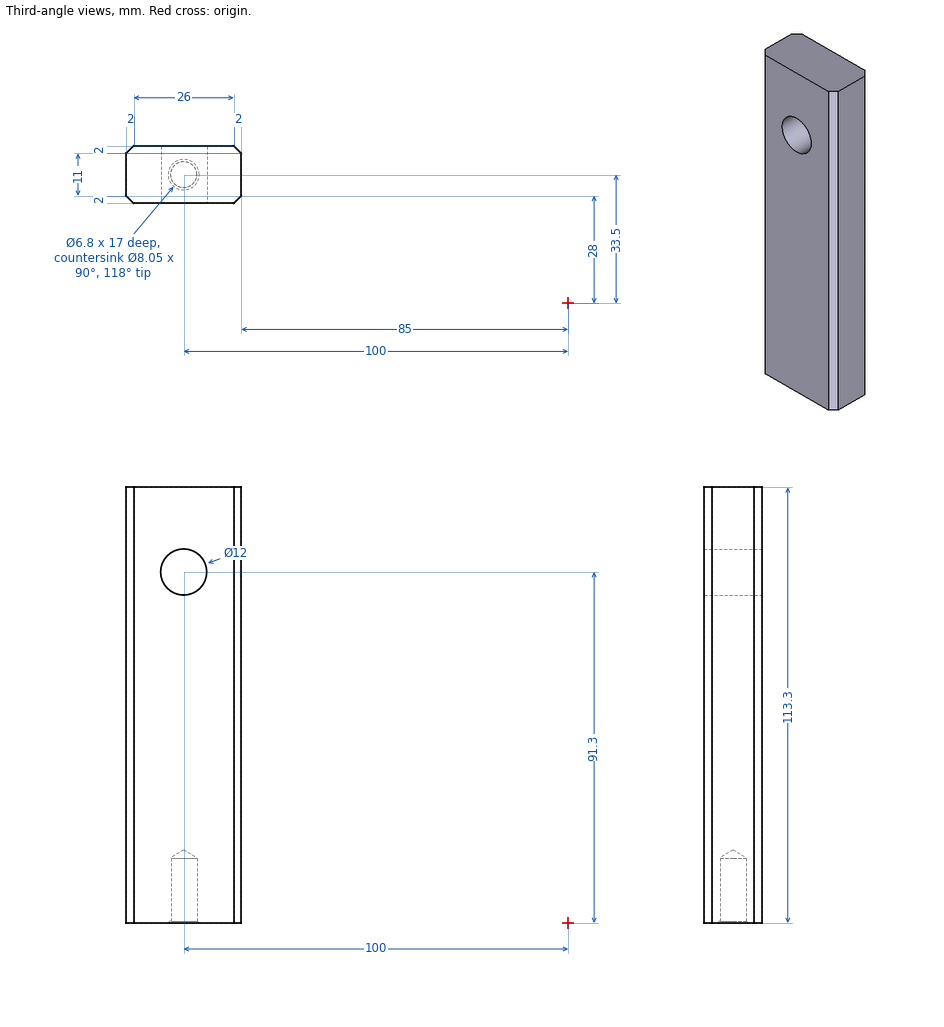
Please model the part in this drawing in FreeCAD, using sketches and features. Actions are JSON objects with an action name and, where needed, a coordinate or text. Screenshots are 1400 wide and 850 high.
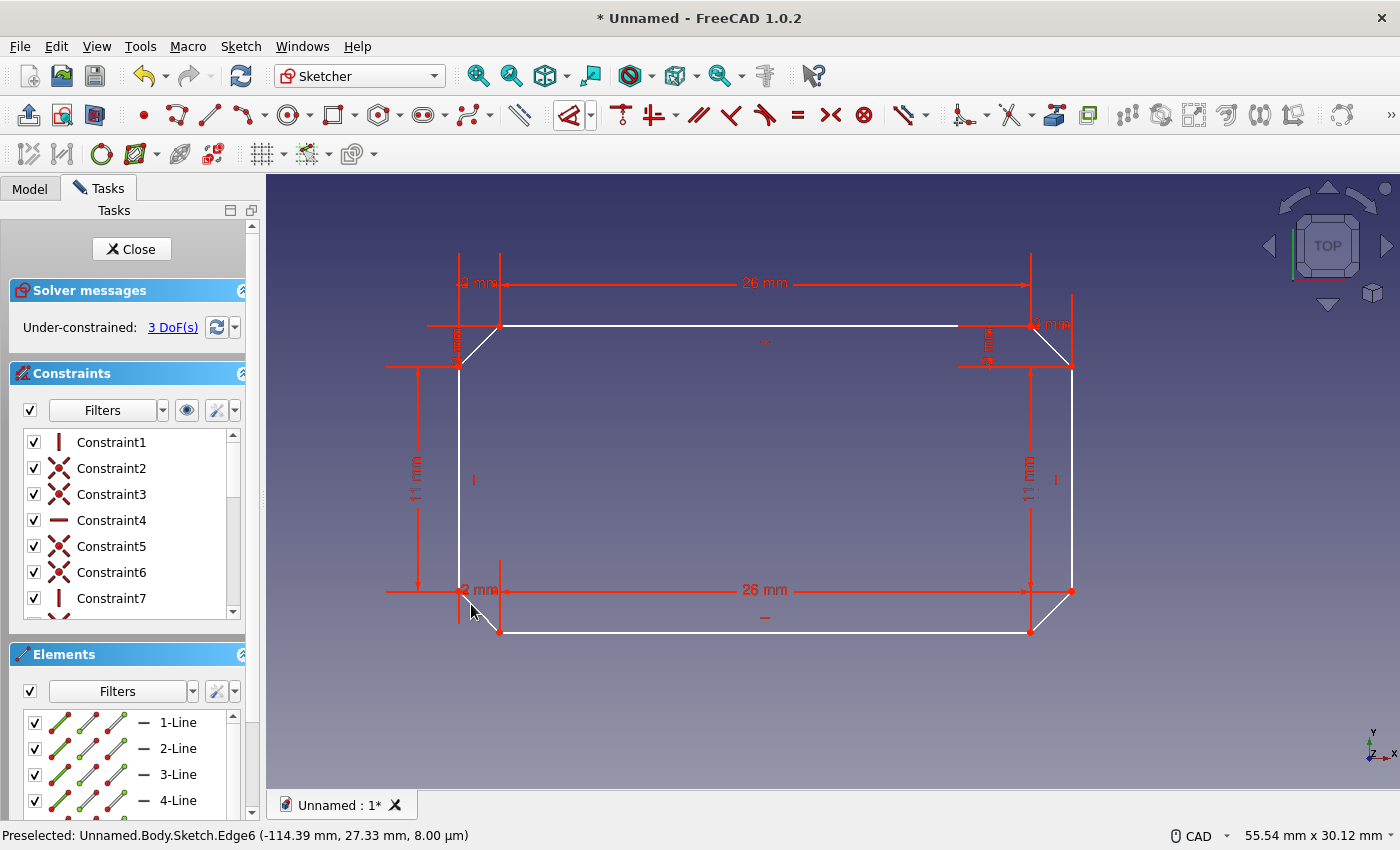
{"action": "left_click", "coordinate": [471, 604]}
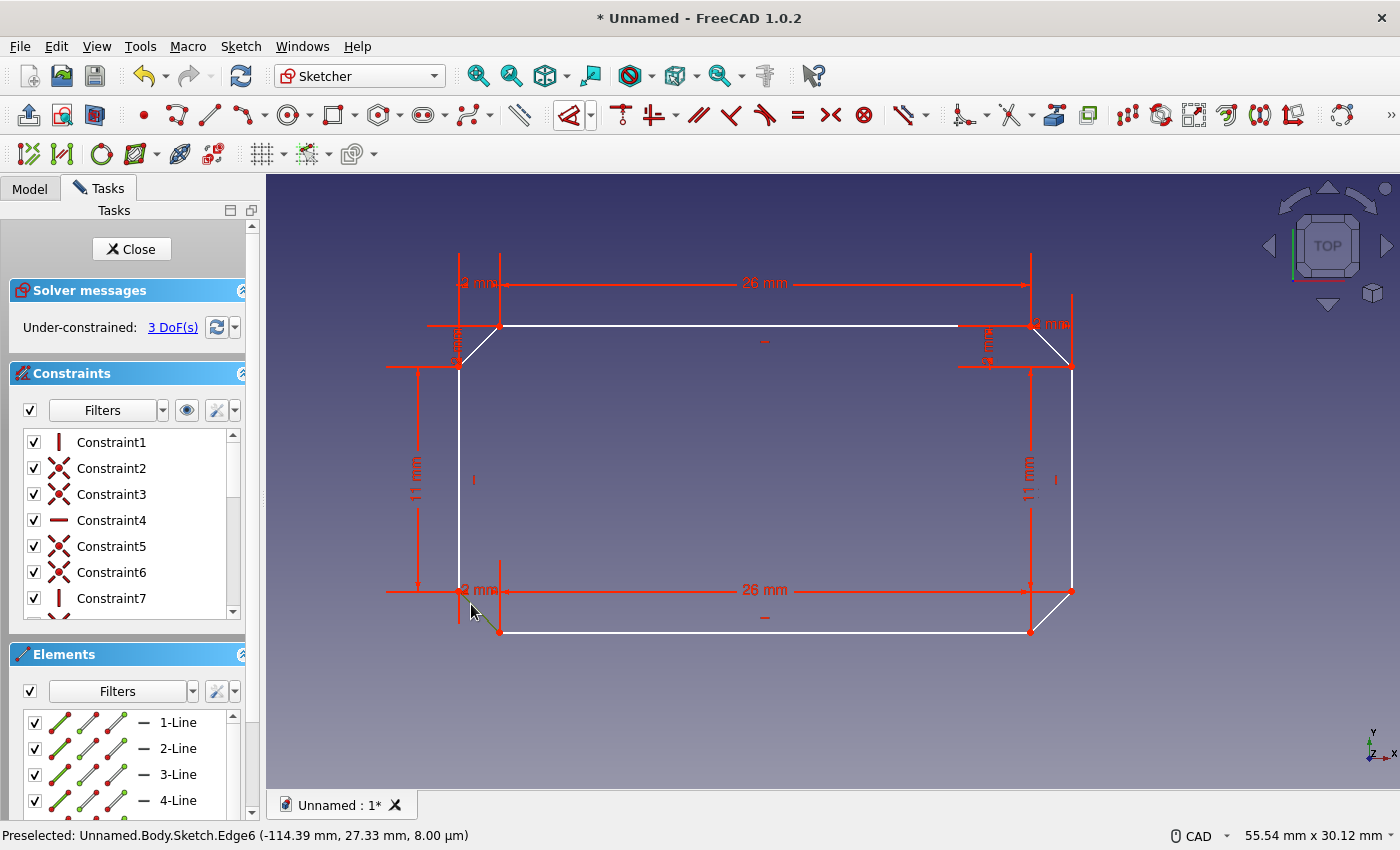
{"action": "left_click", "coordinate": [590, 116]}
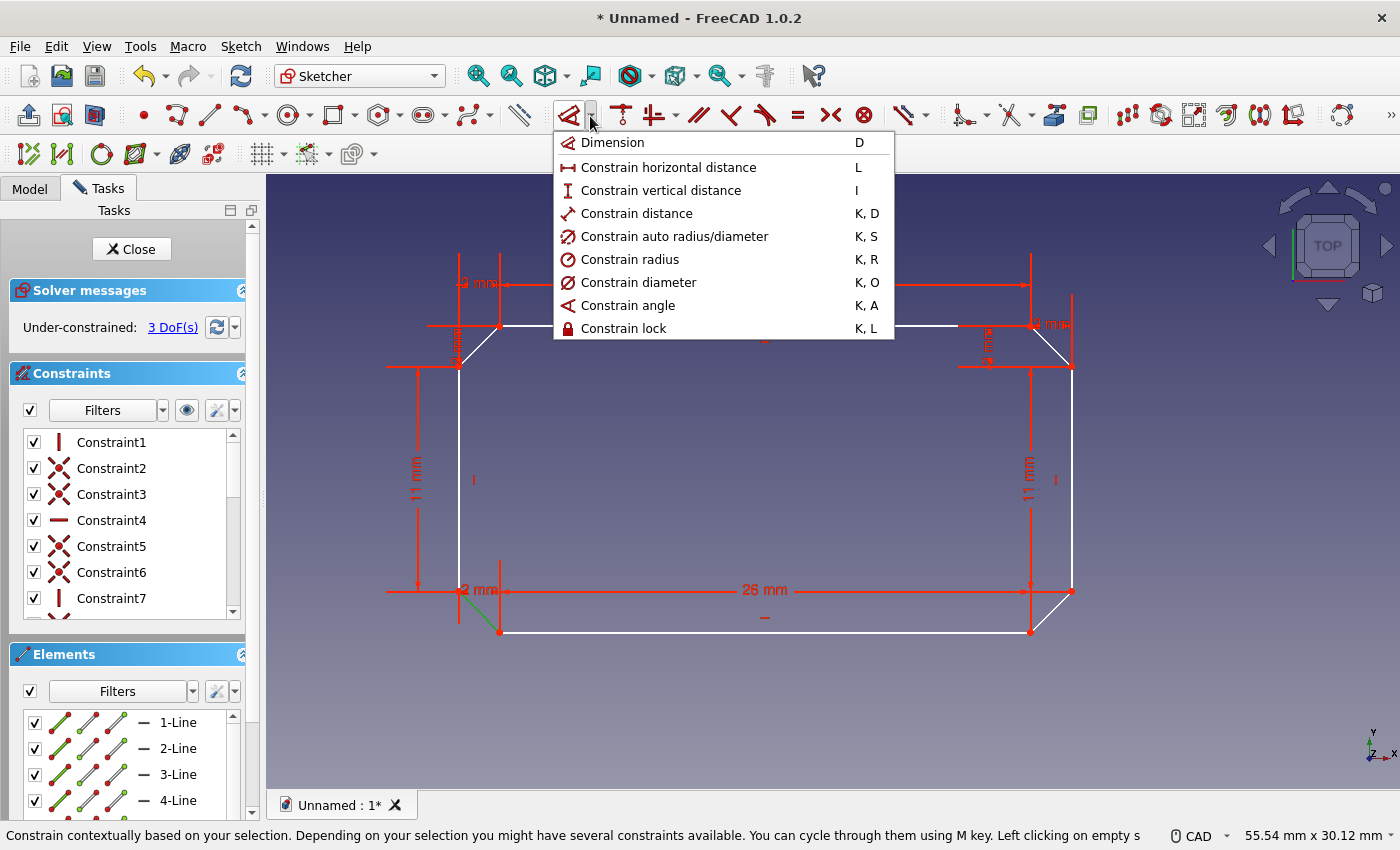
{"action": "left_click", "coordinate": [724, 190]}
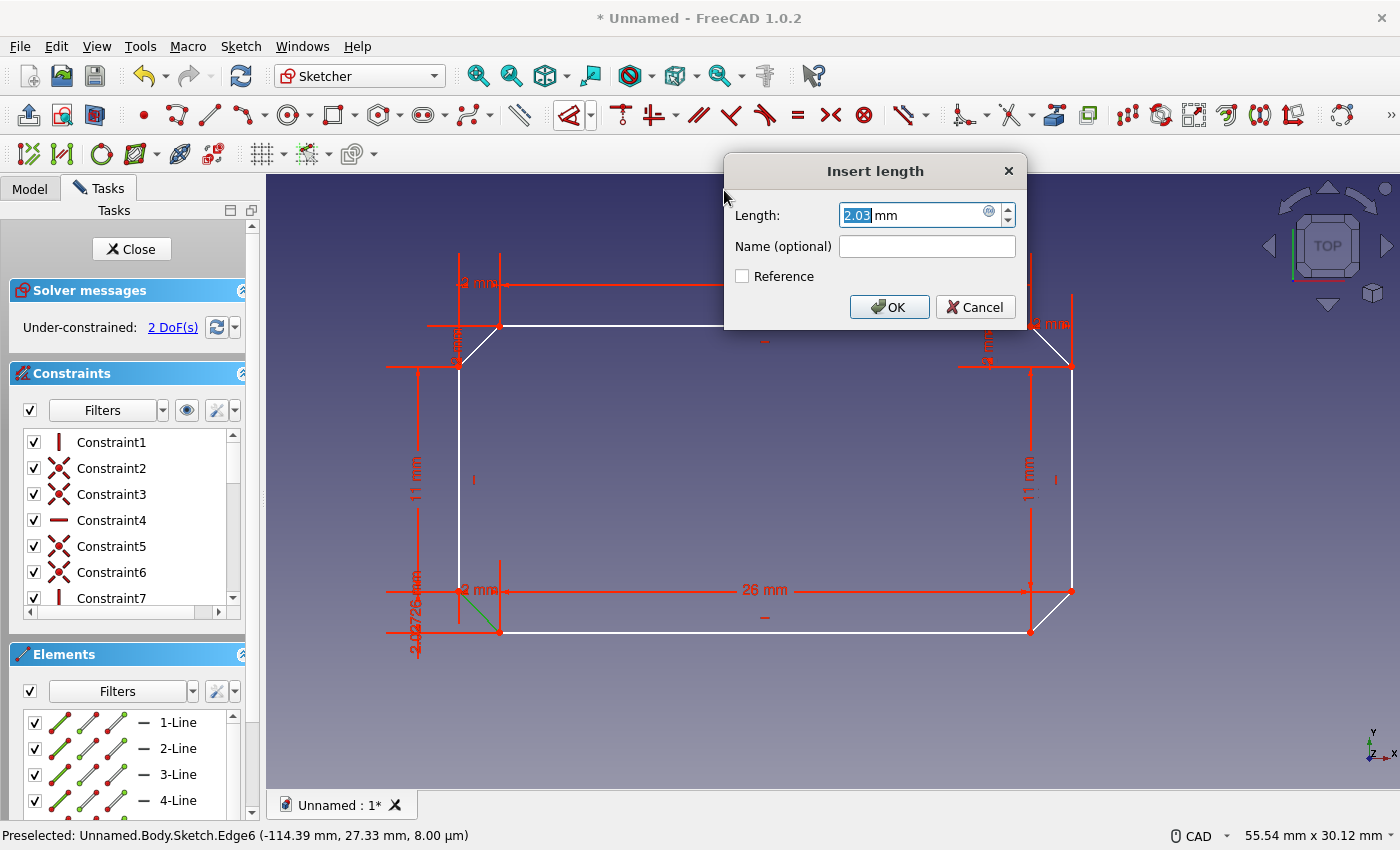
{"action": "type", "text": "2"}
{"action": "key", "text": "Return"}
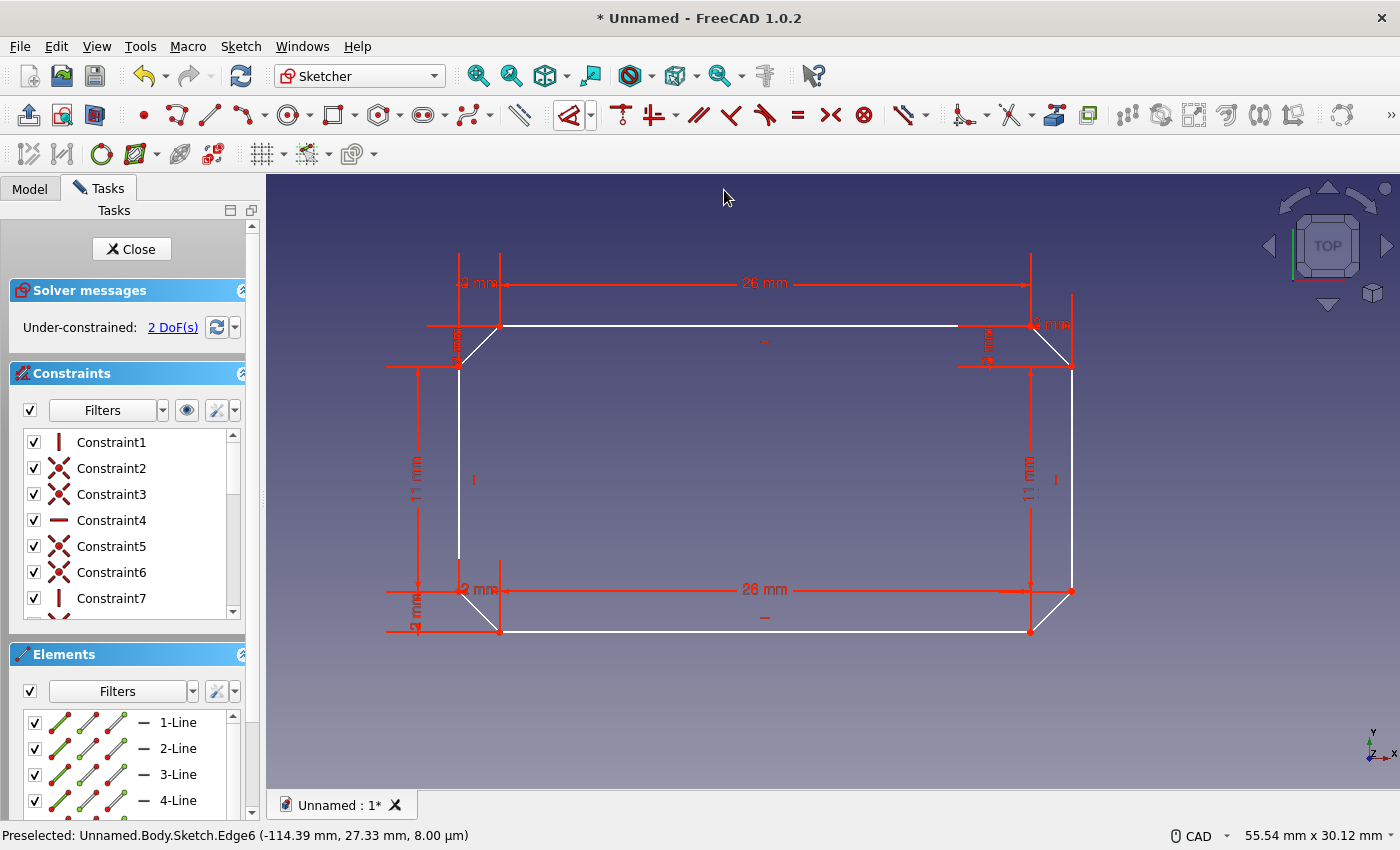
{"action": "left_click", "coordinate": [1072, 592]}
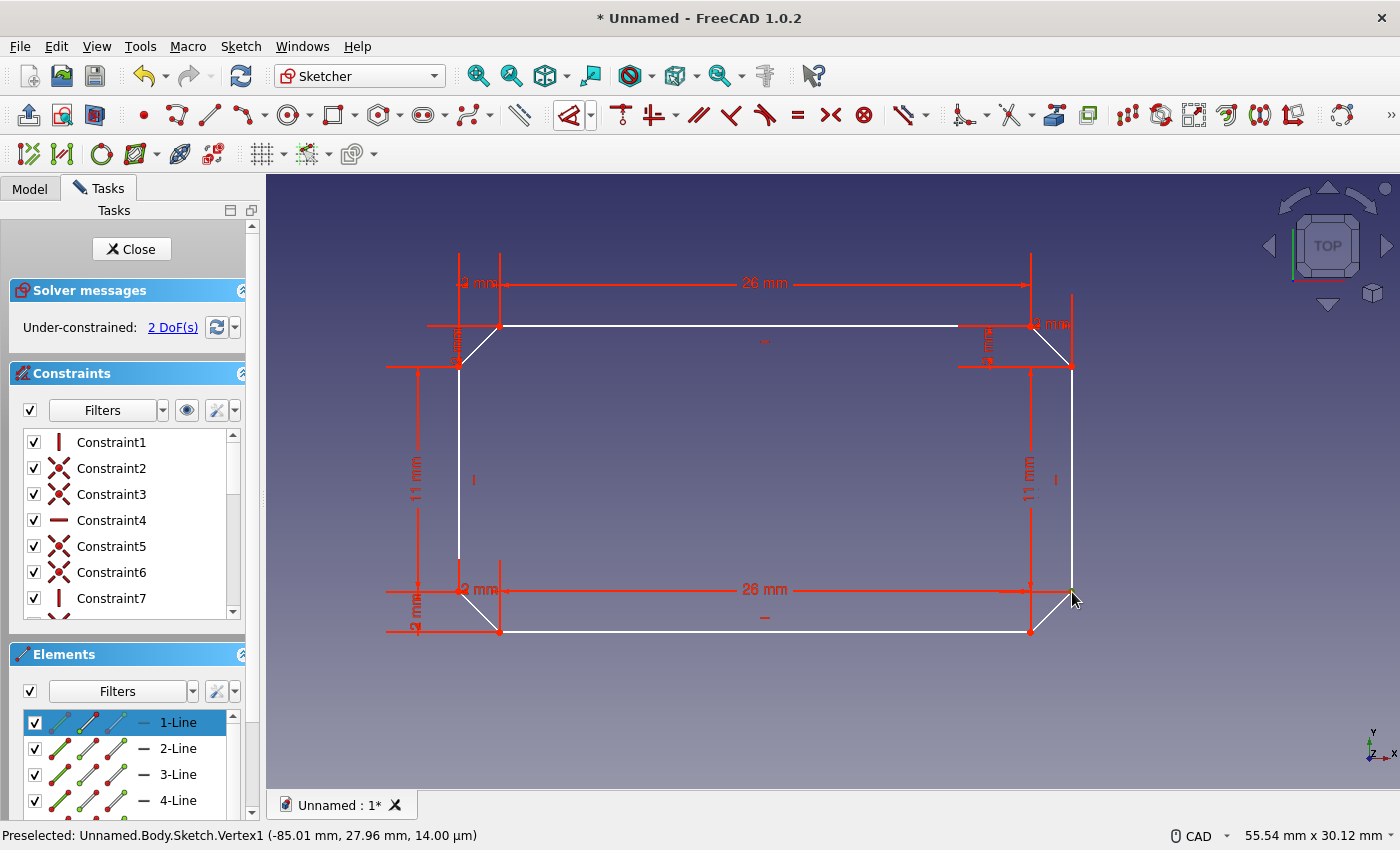
{"action": "left_click", "coordinate": [590, 116]}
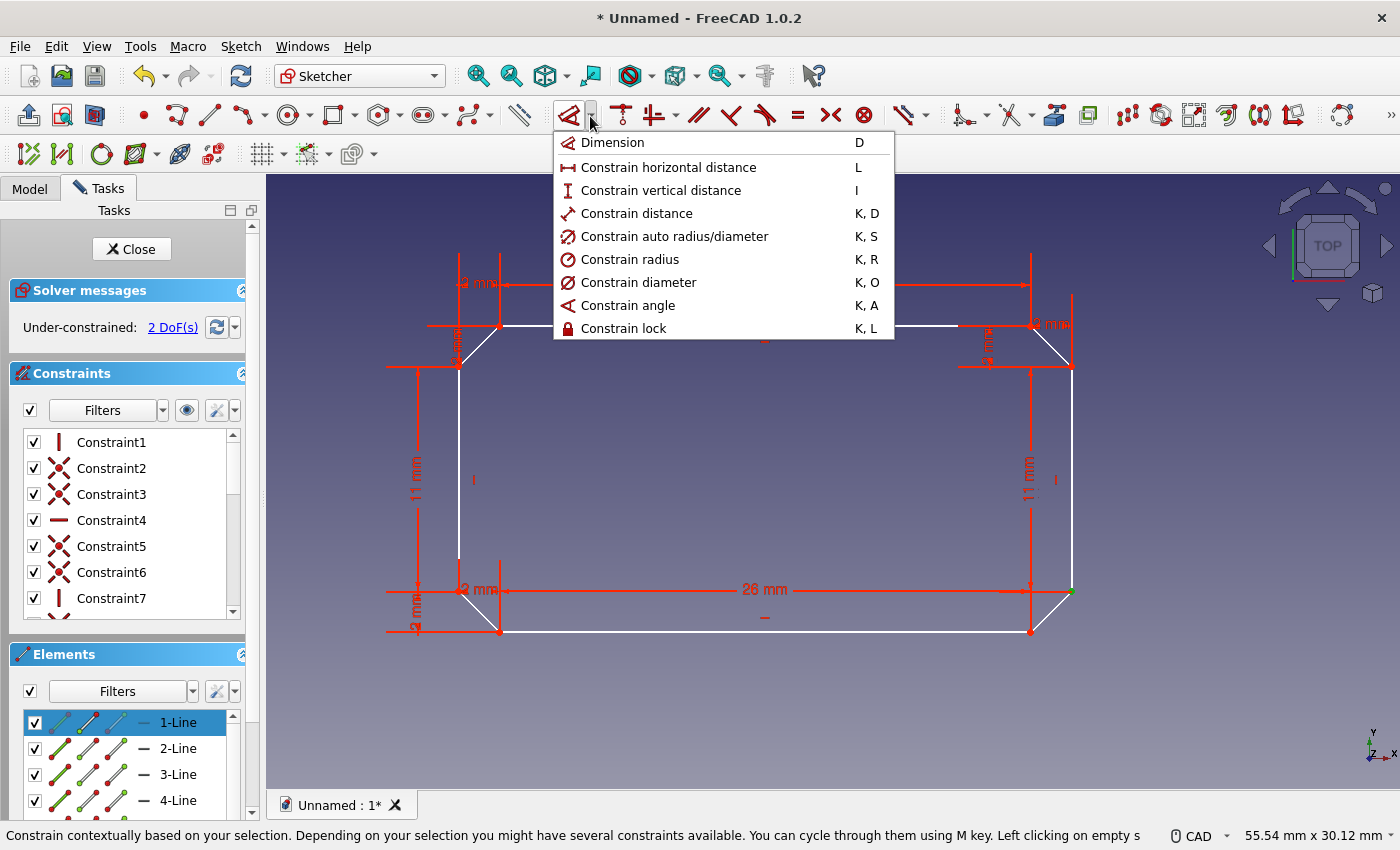
{"action": "left_click", "coordinate": [724, 168]}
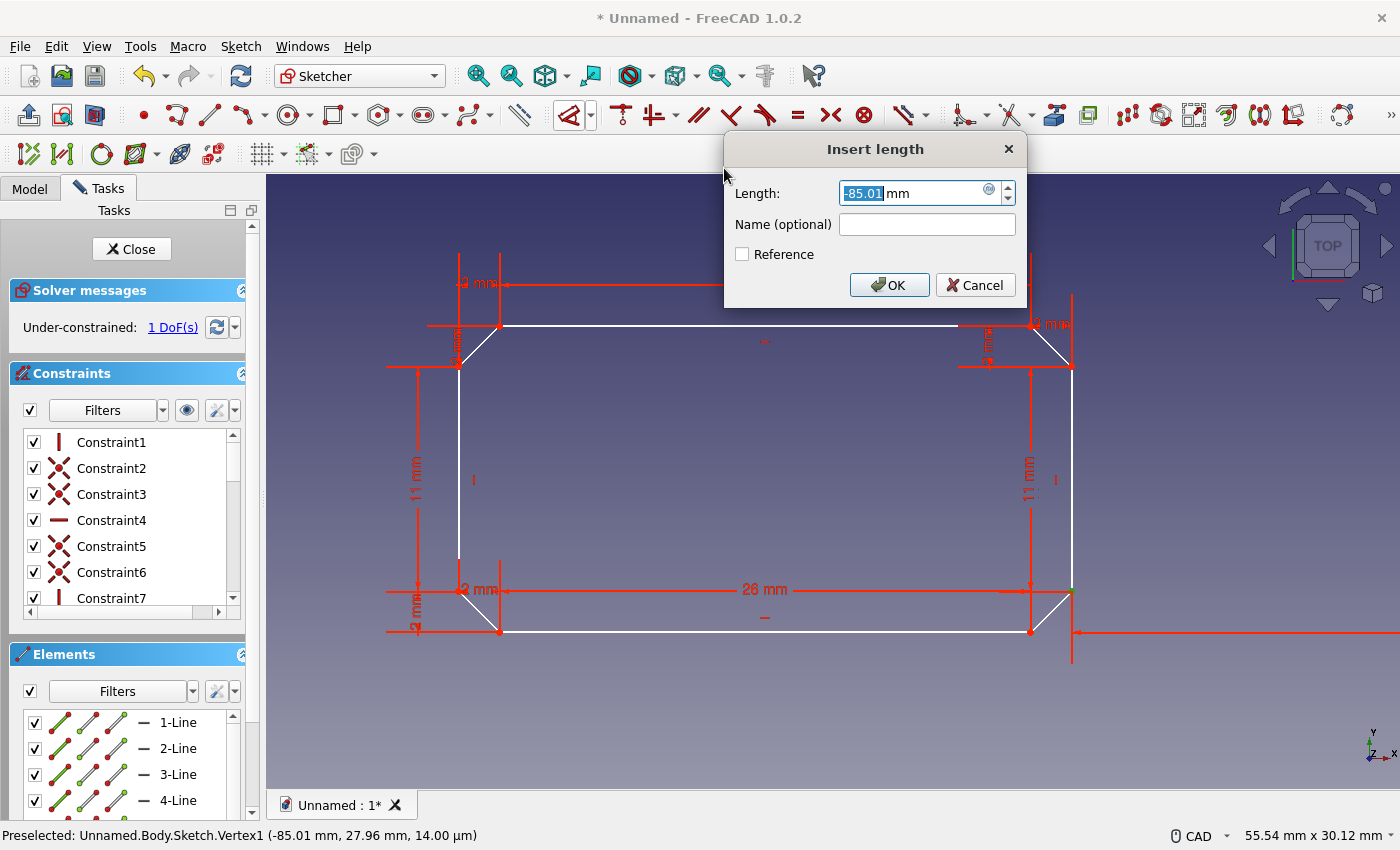
{"action": "type", "text": "-85"}
{"action": "key", "text": "Return"}